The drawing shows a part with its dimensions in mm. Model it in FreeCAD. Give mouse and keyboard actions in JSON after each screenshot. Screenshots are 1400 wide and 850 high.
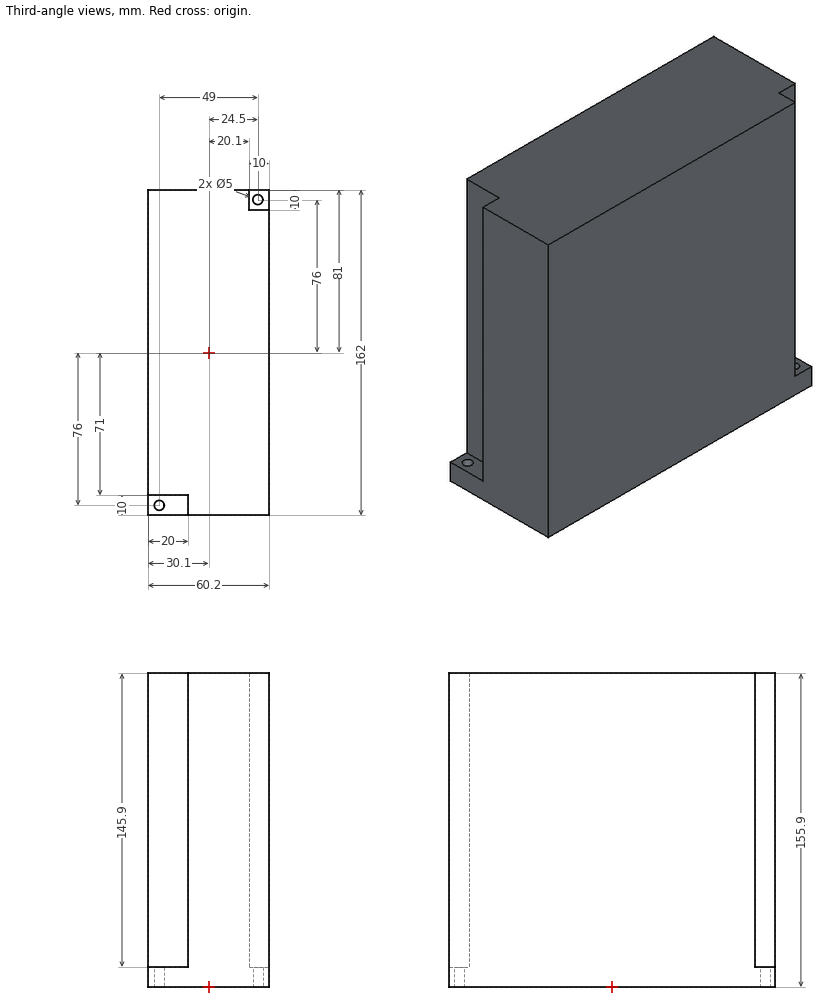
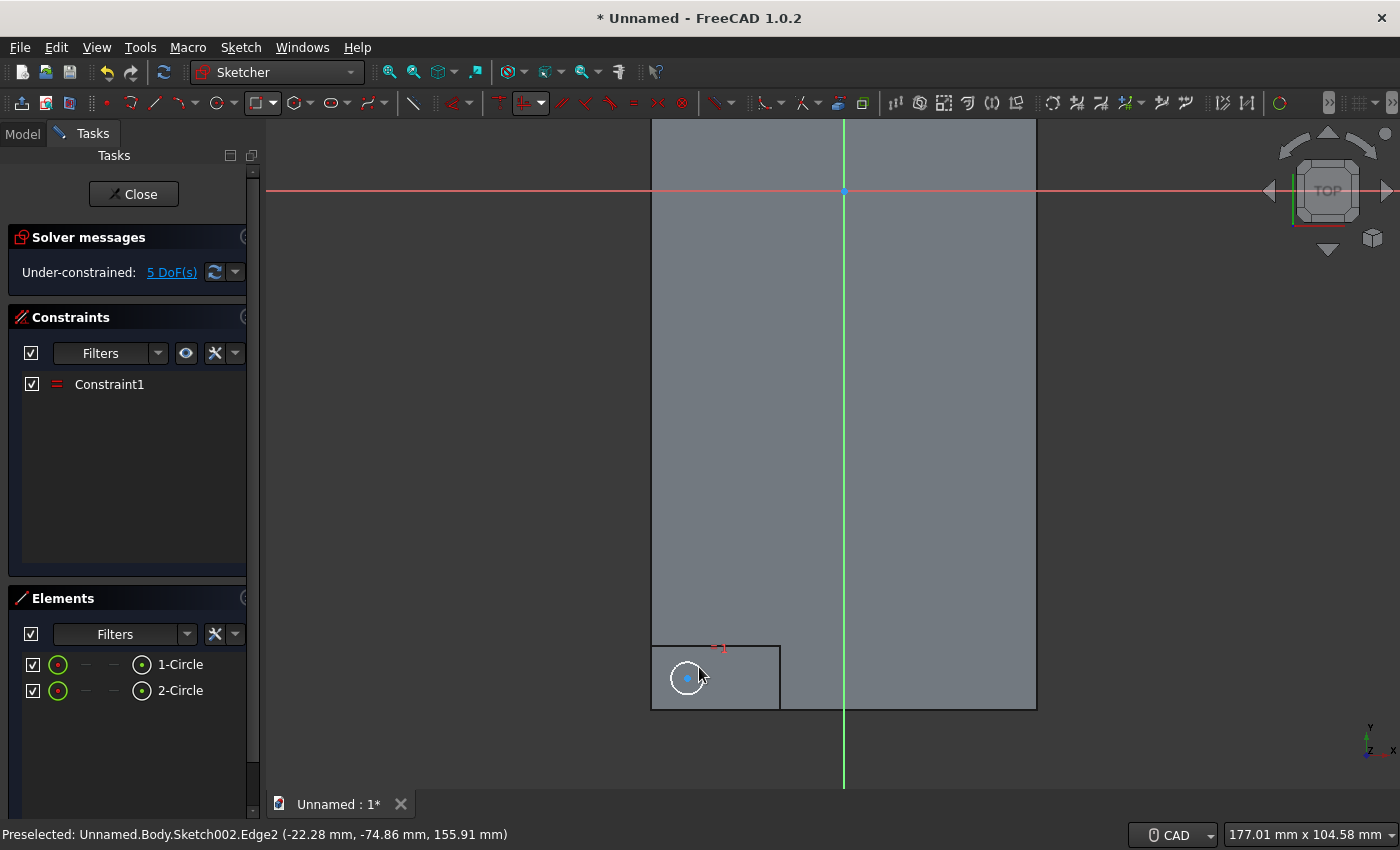
{"action": "key", "text": "d"}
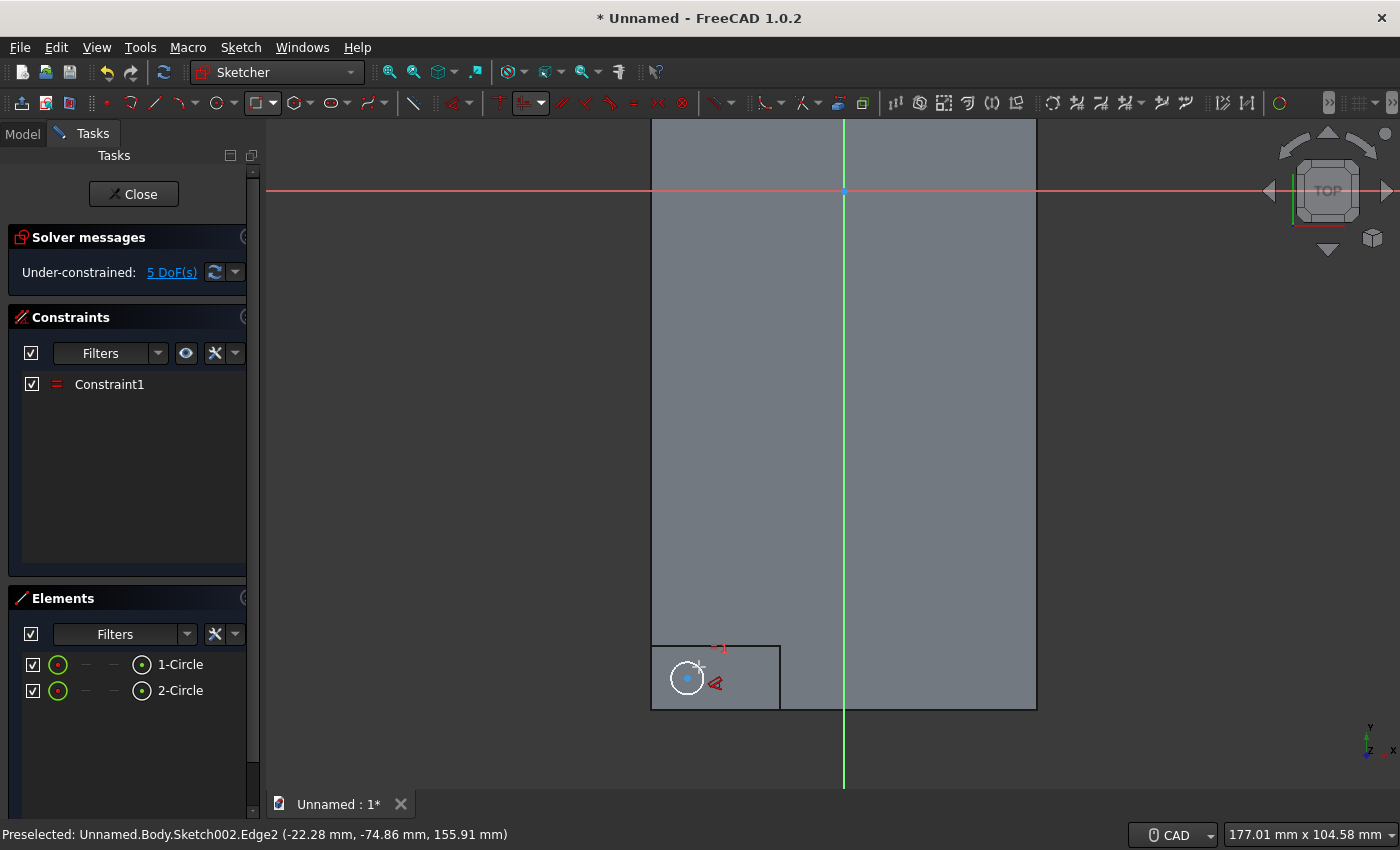
{"action": "scroll", "coordinate": [699, 669], "scroll_direction": "down", "scroll_amount": 4}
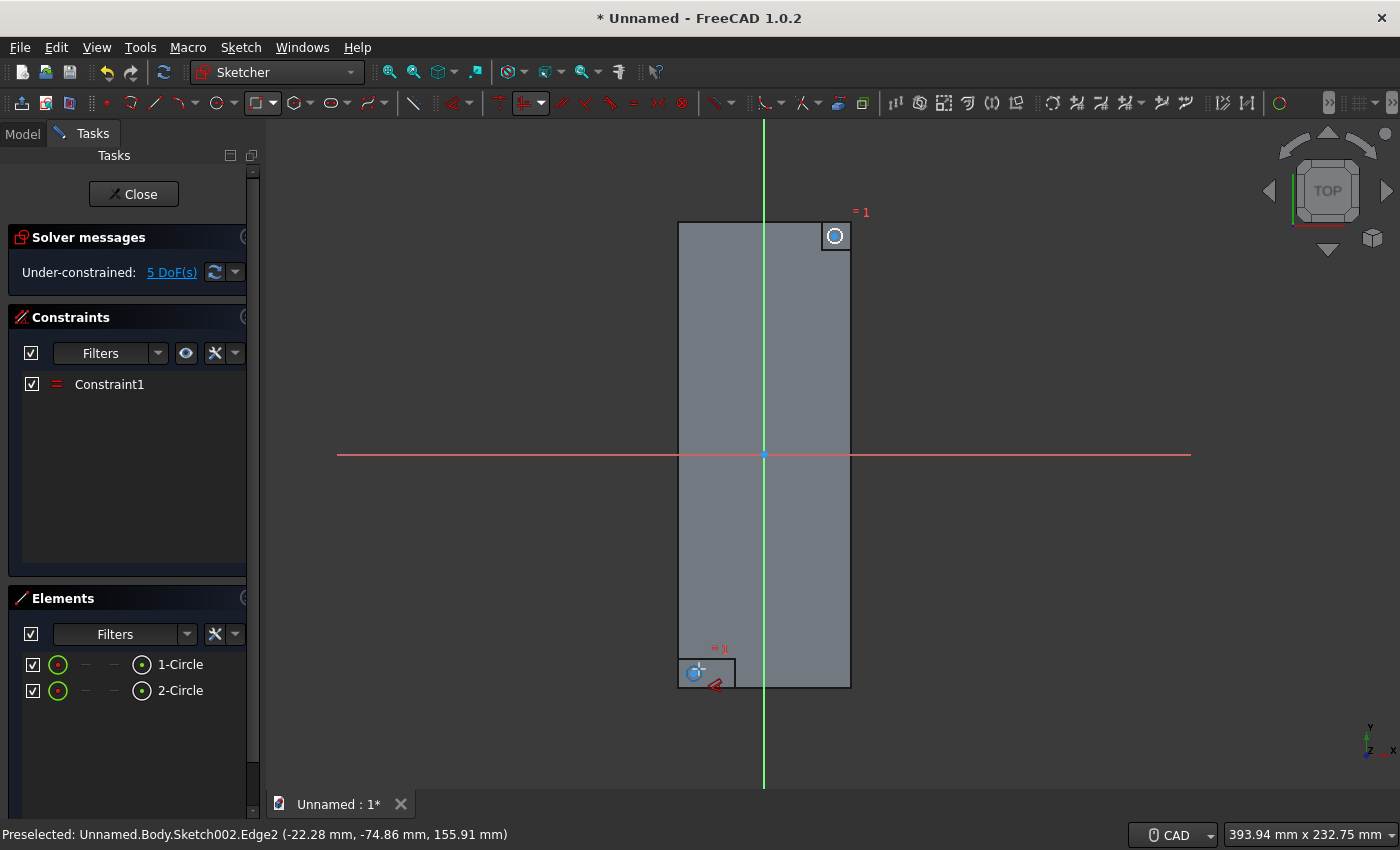
{"action": "scroll", "coordinate": [840, 231], "scroll_direction": "up", "scroll_amount": 6}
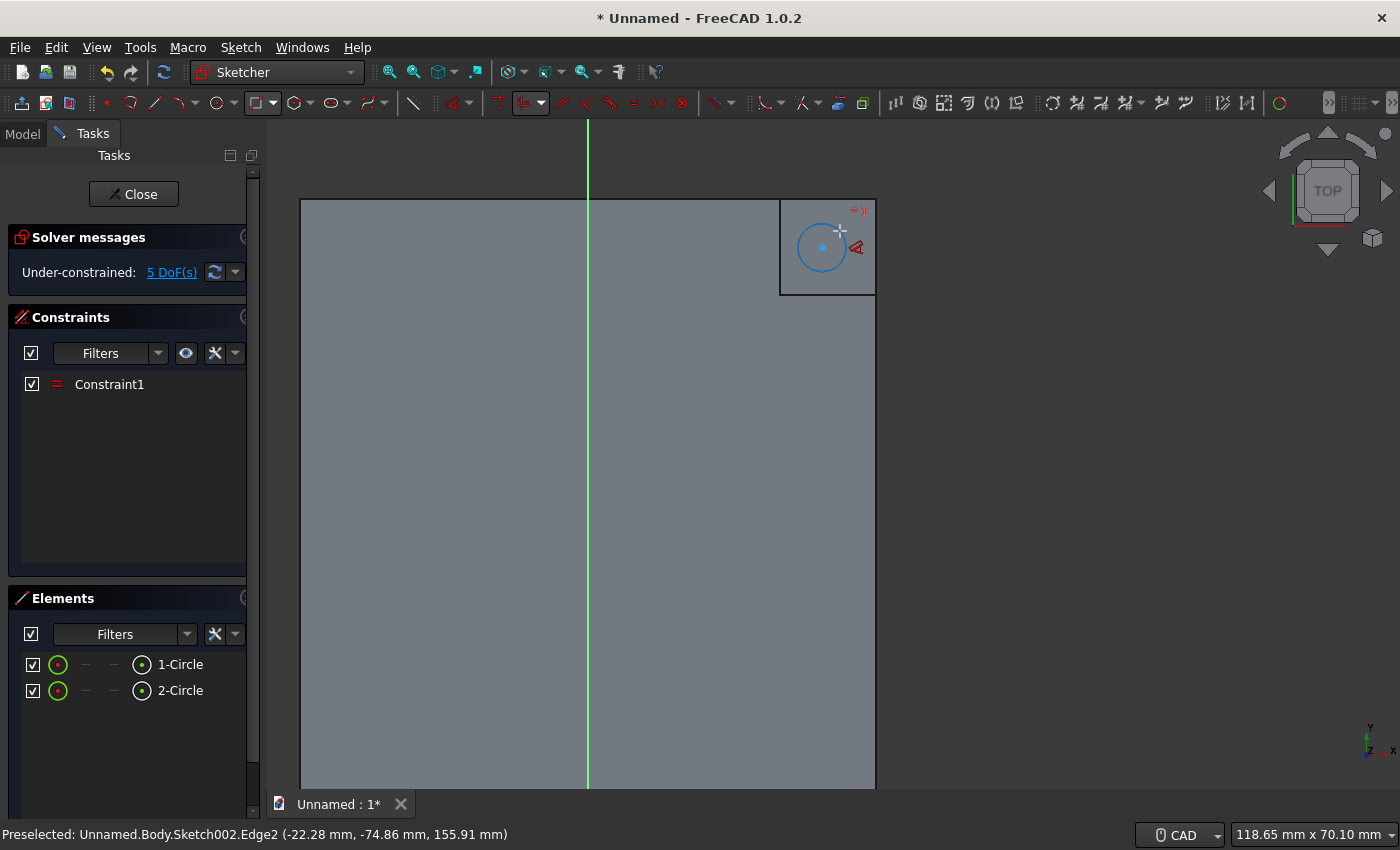
{"action": "left_click", "coordinate": [839, 231]}
{"action": "left_click", "coordinate": [862, 209]}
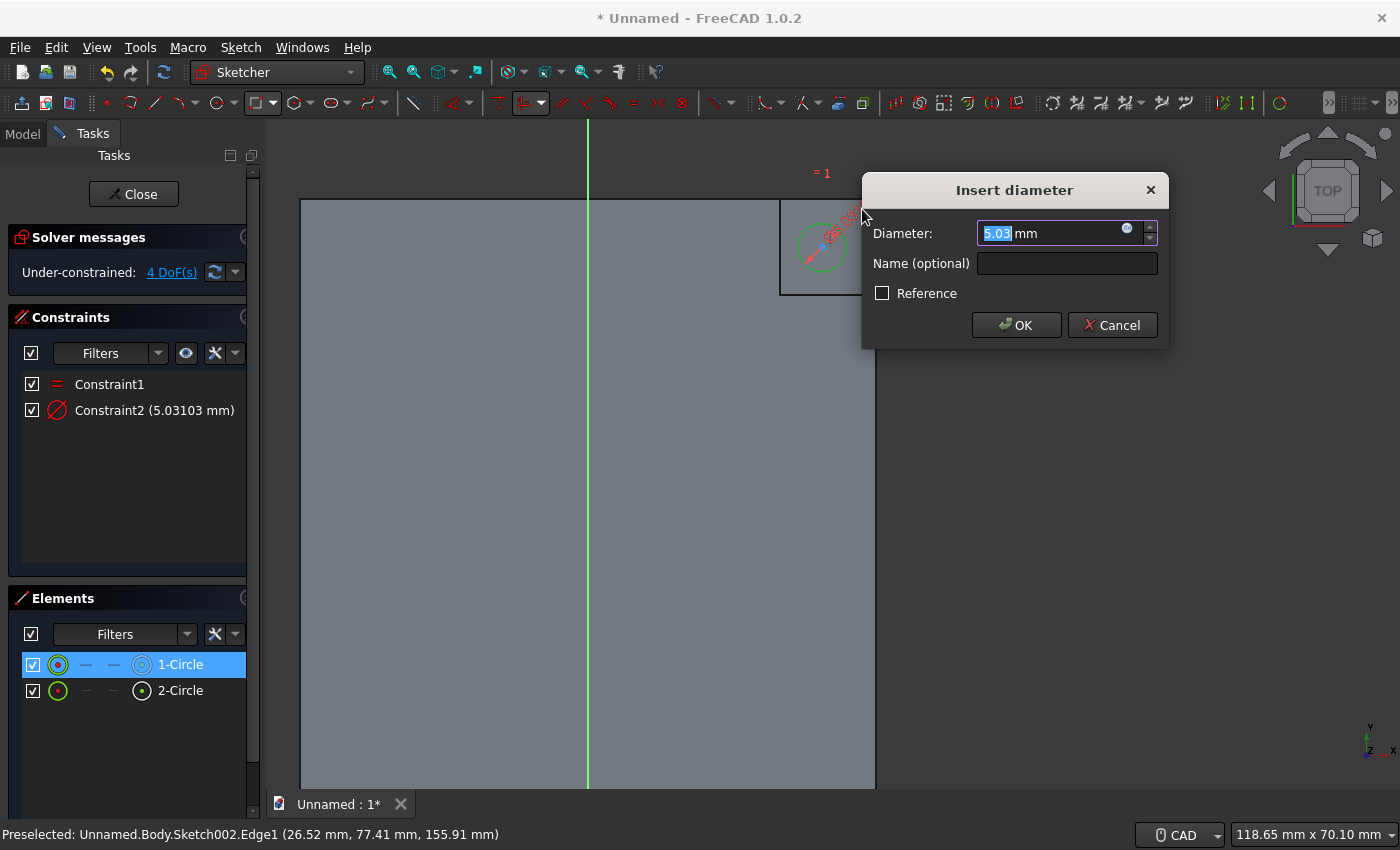
{"action": "type", "text": "5"}
{"action": "key", "text": "Return"}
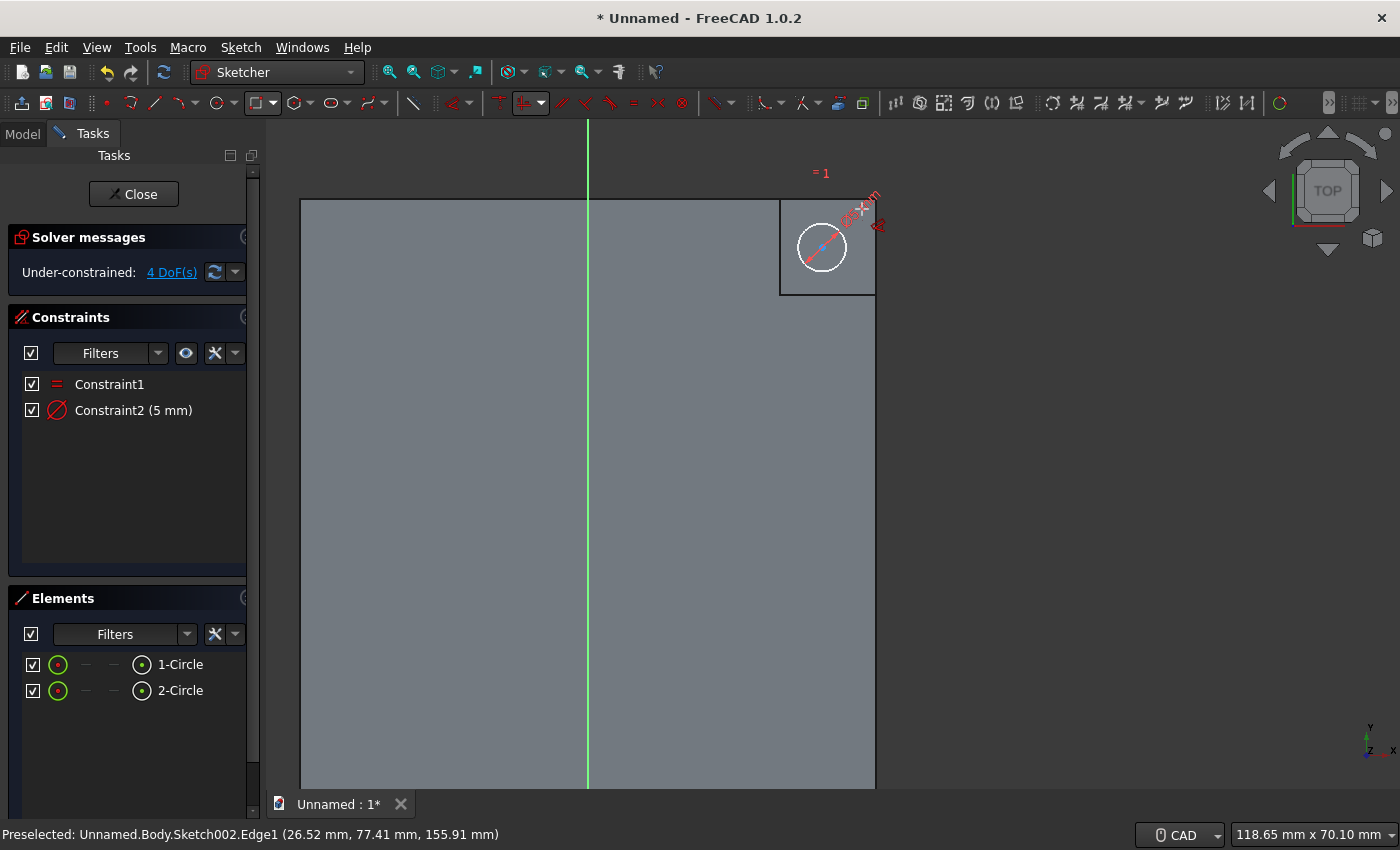
{"action": "left_click", "coordinate": [822, 248]}
{"action": "left_click", "coordinate": [856, 504]}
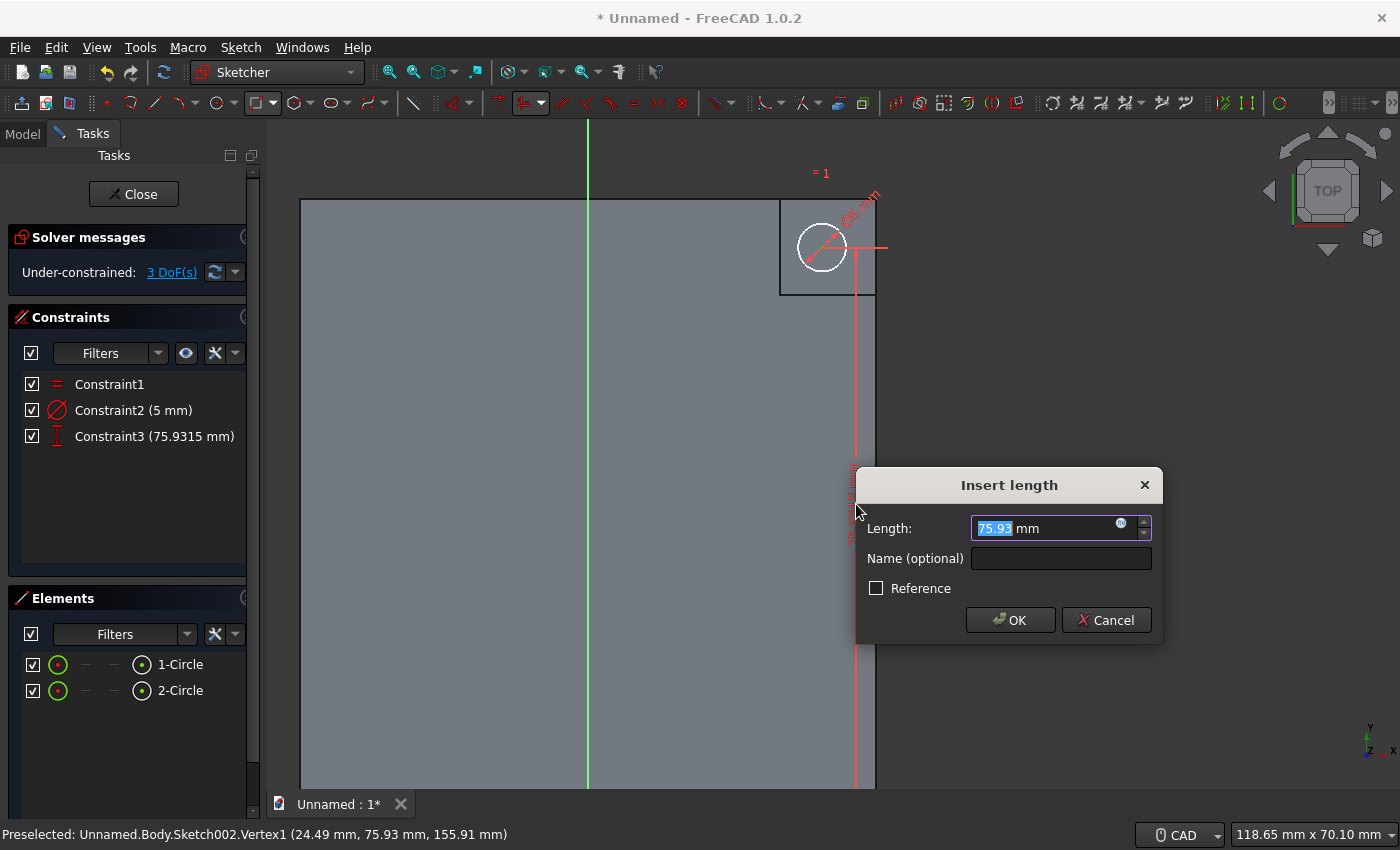
{"action": "type", "text": "76"}
{"action": "key", "text": "Return"}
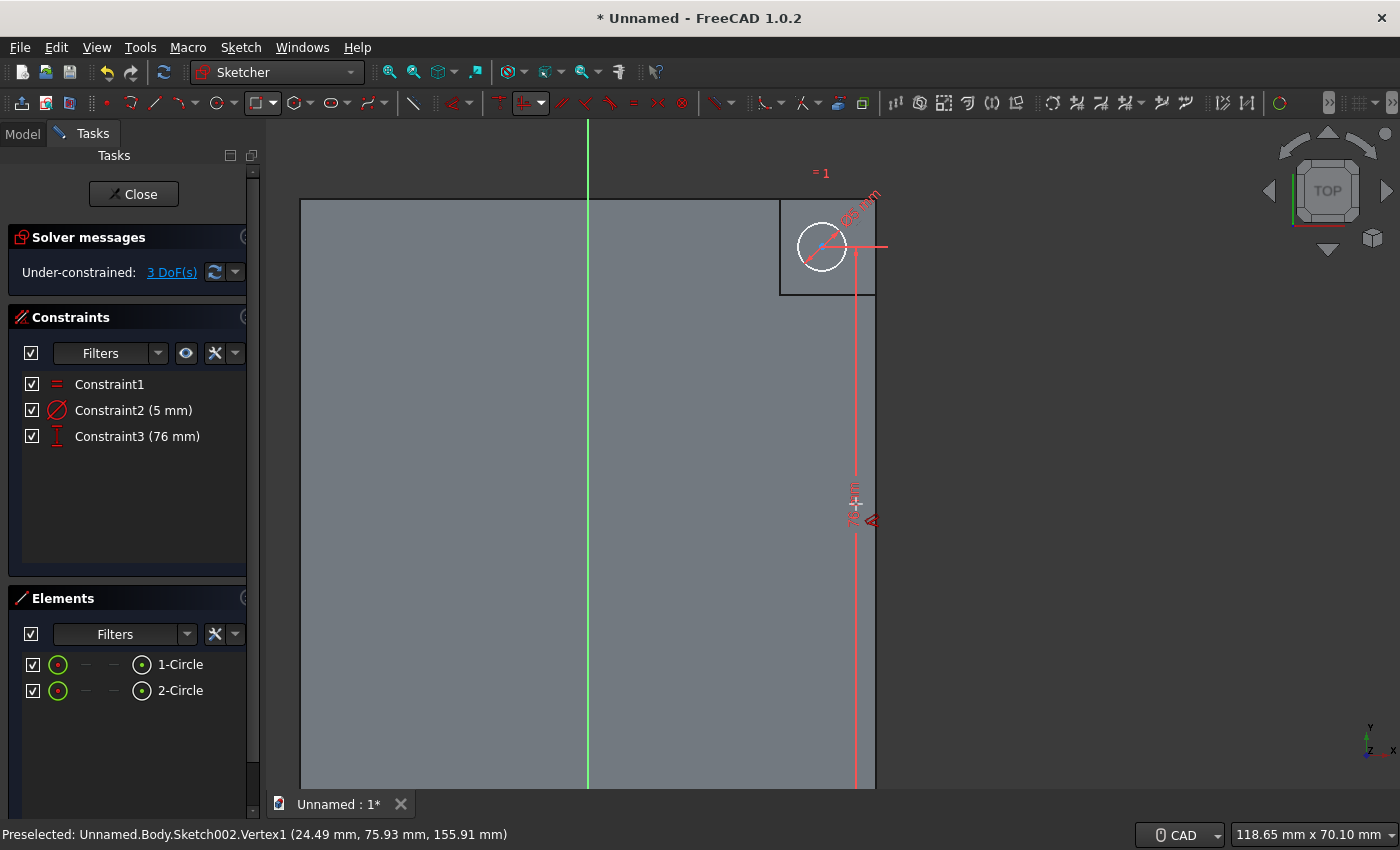
{"action": "scroll", "coordinate": [841, 230], "scroll_direction": "down", "scroll_amount": 6}